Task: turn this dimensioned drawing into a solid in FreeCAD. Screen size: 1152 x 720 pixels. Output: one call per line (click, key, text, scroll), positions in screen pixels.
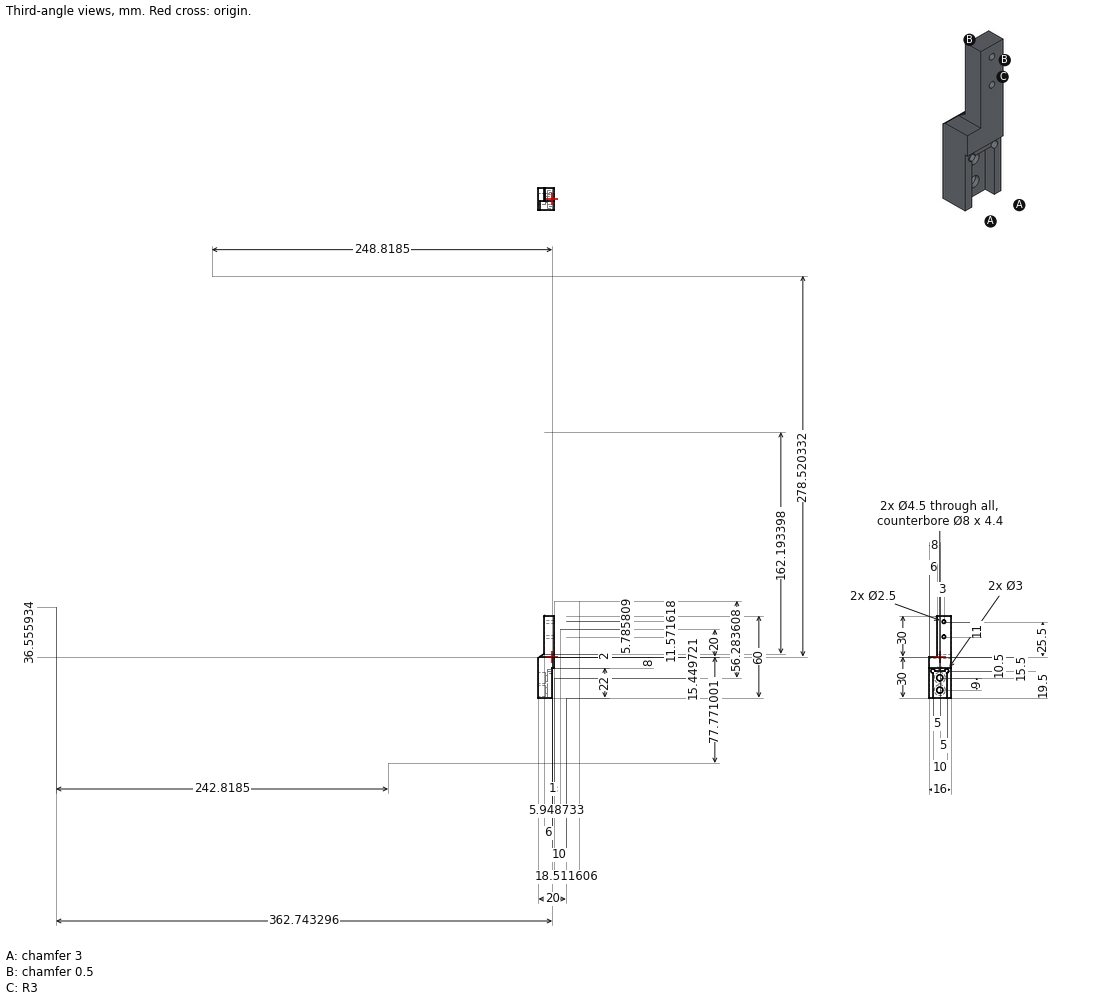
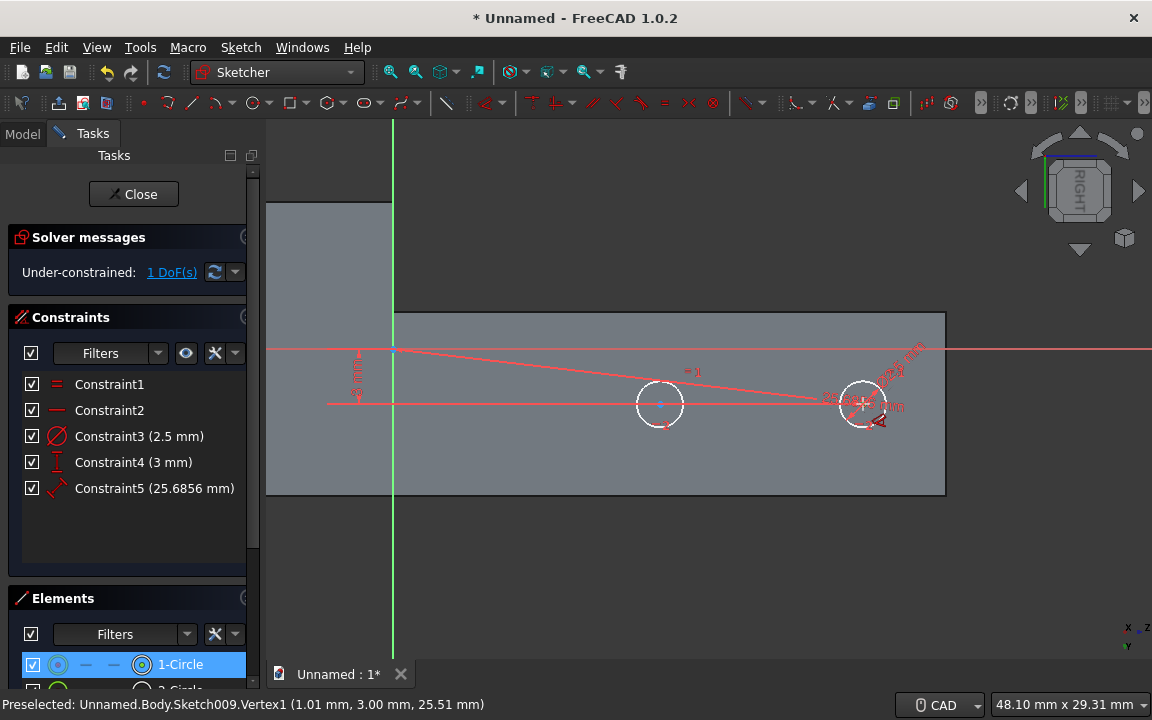
click(660, 404)
click(762, 438)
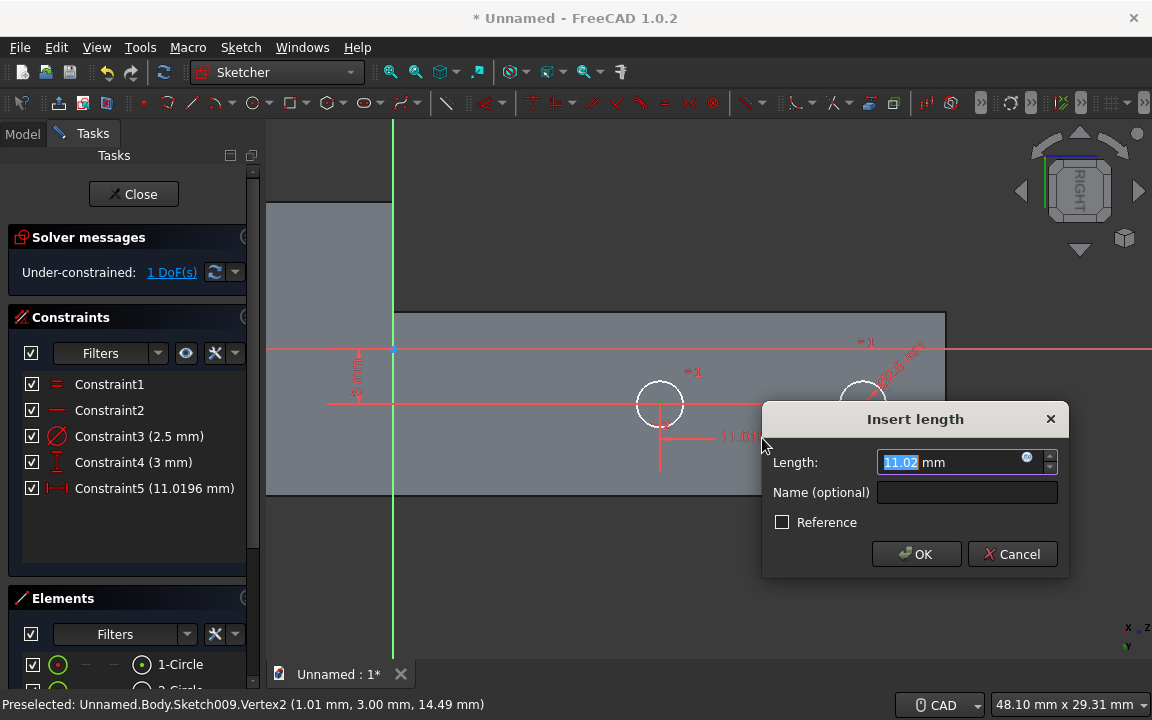
text(11)
key(Return)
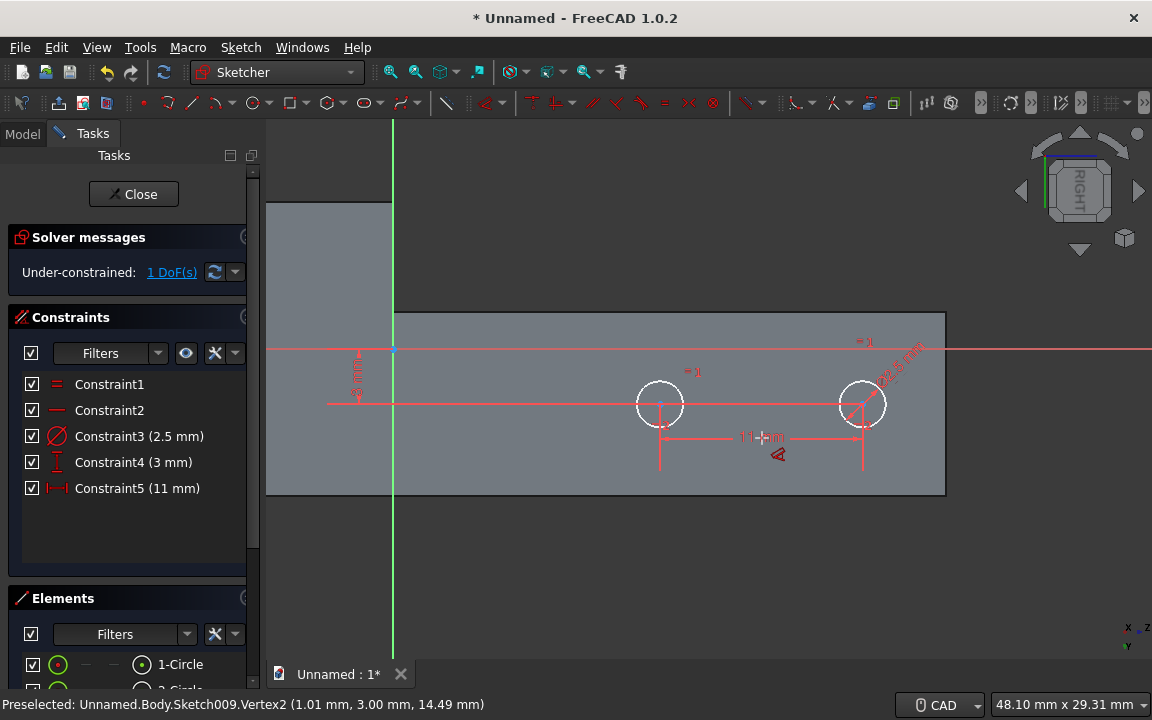
click(863, 404)
click(628, 315)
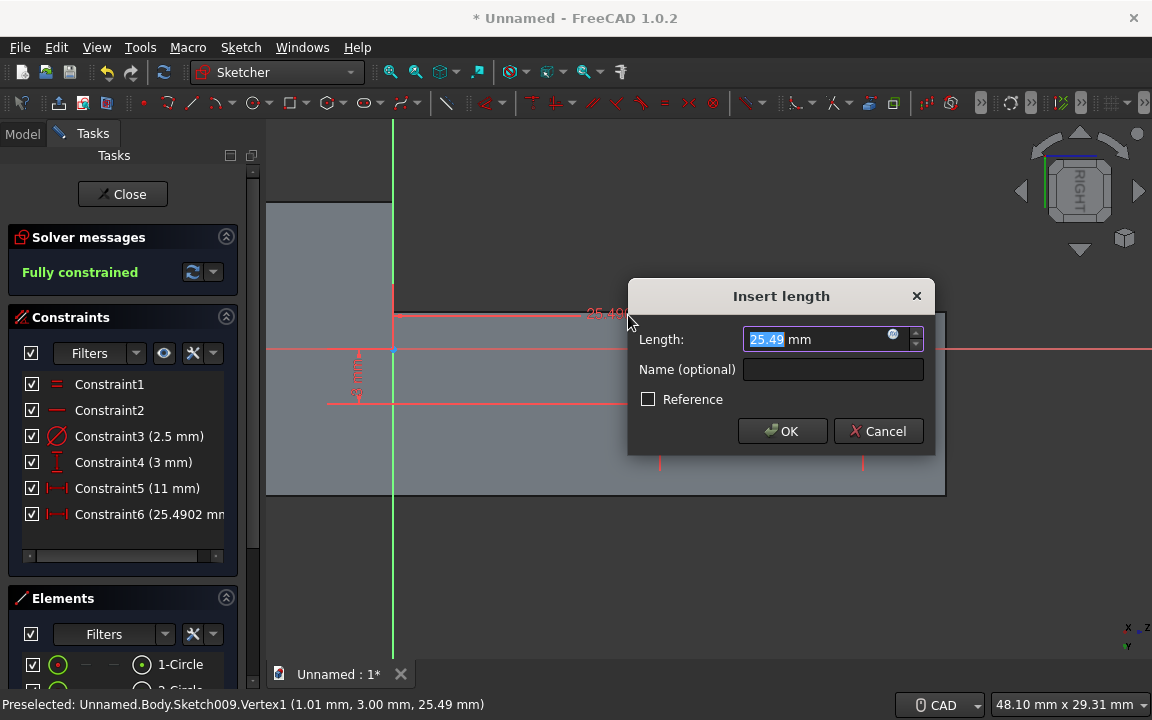
text(25.5)
key(Return)
key(Escape)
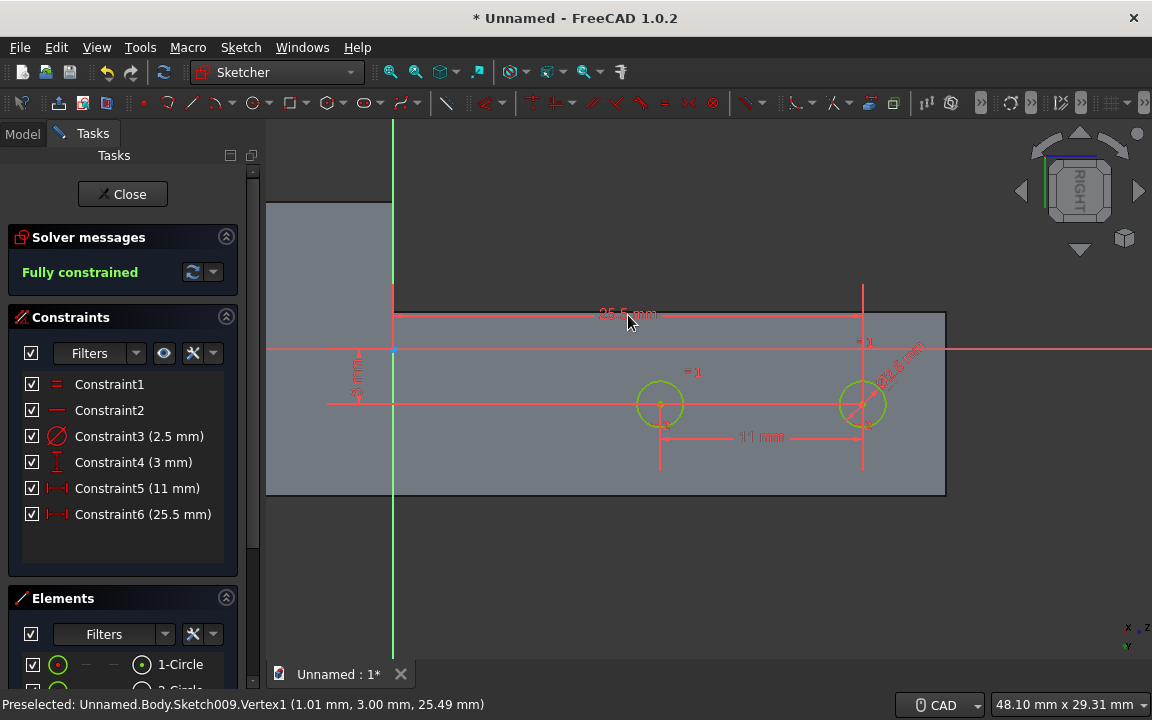
click(123, 194)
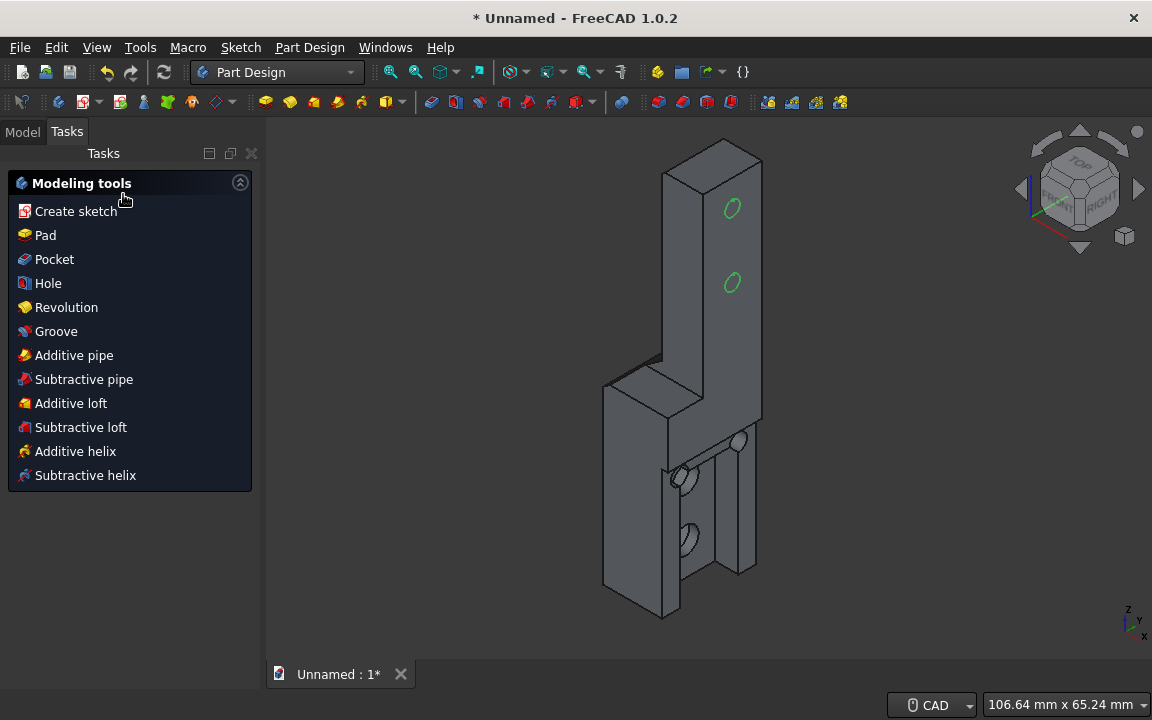
click(432, 102)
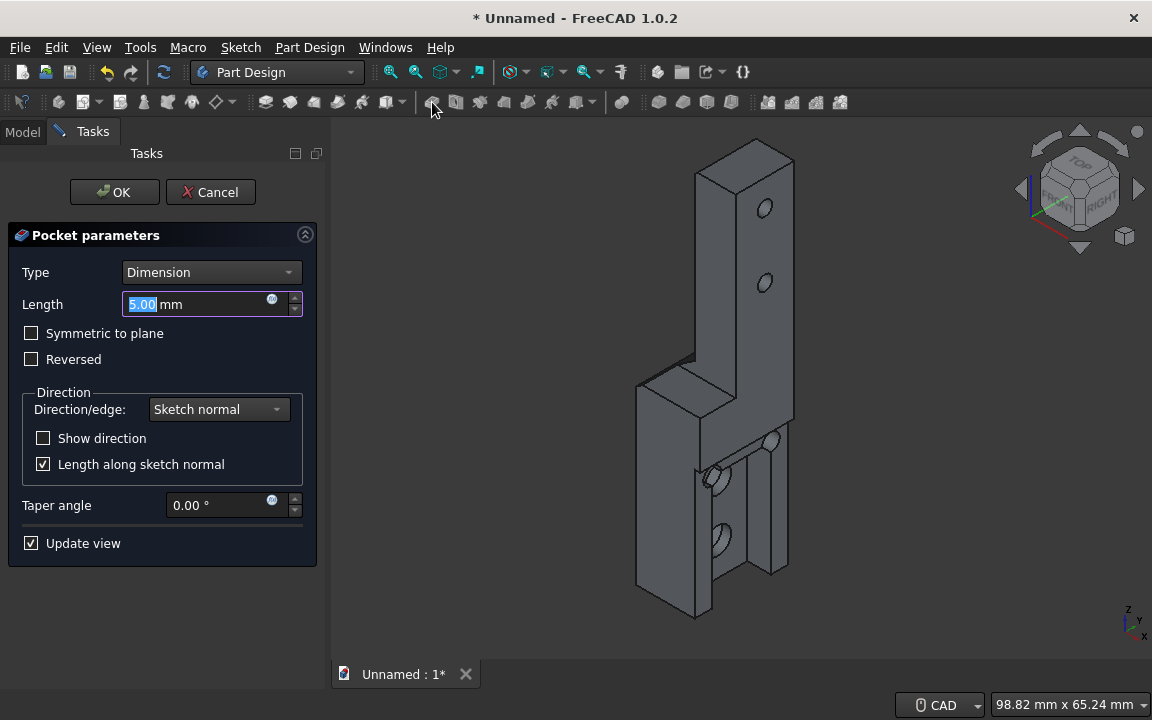
click(212, 272)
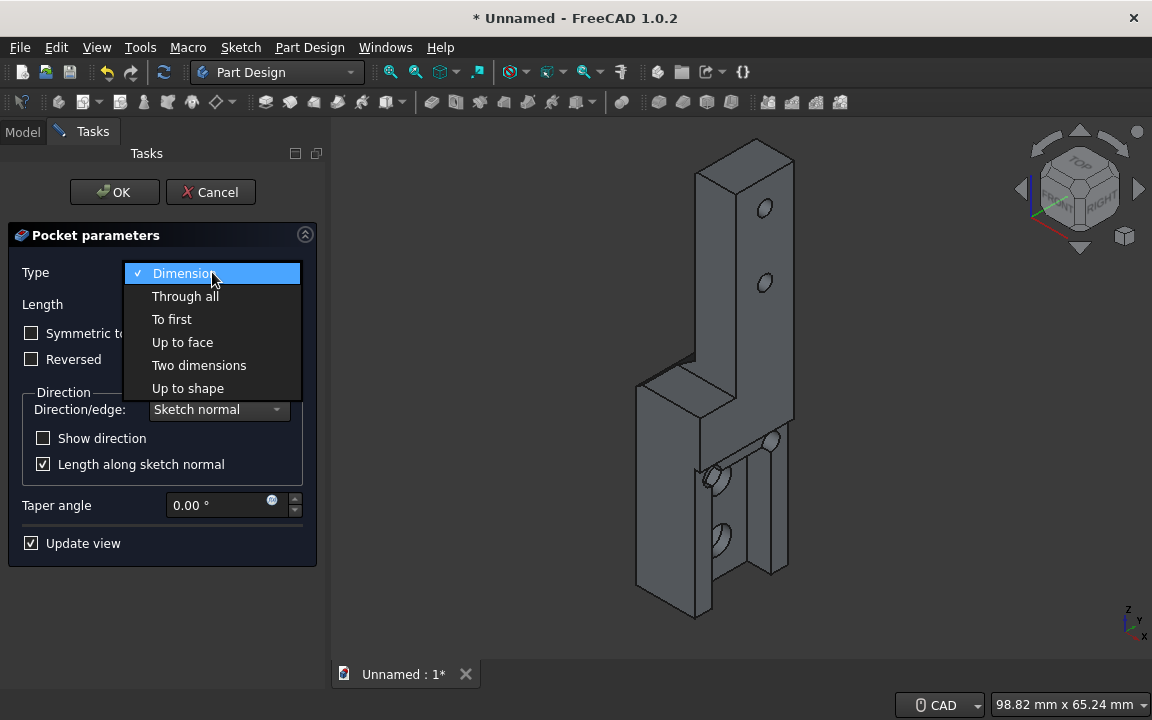
click(212, 296)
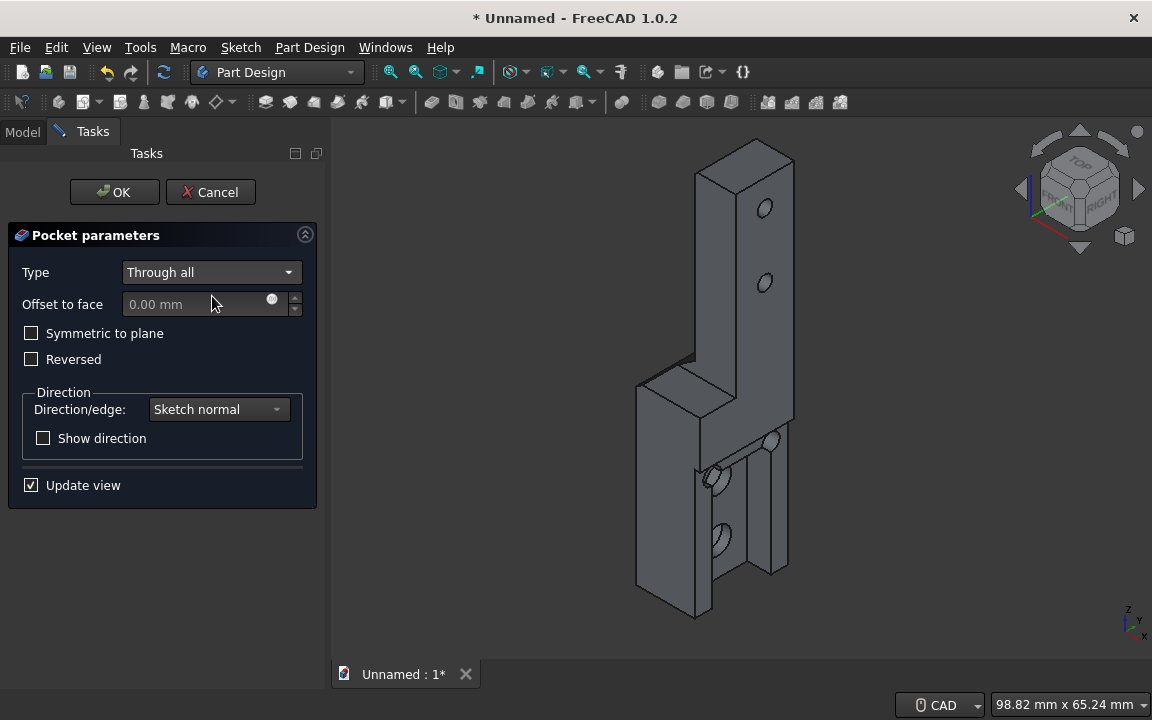
click(115, 192)